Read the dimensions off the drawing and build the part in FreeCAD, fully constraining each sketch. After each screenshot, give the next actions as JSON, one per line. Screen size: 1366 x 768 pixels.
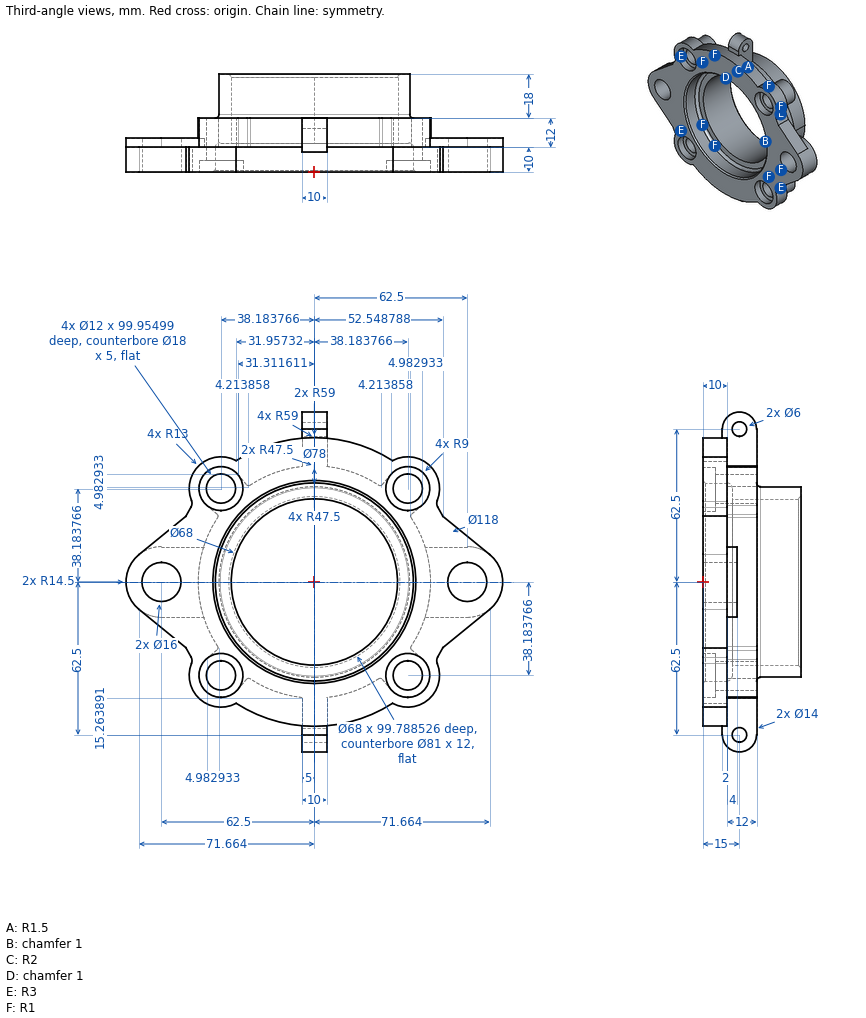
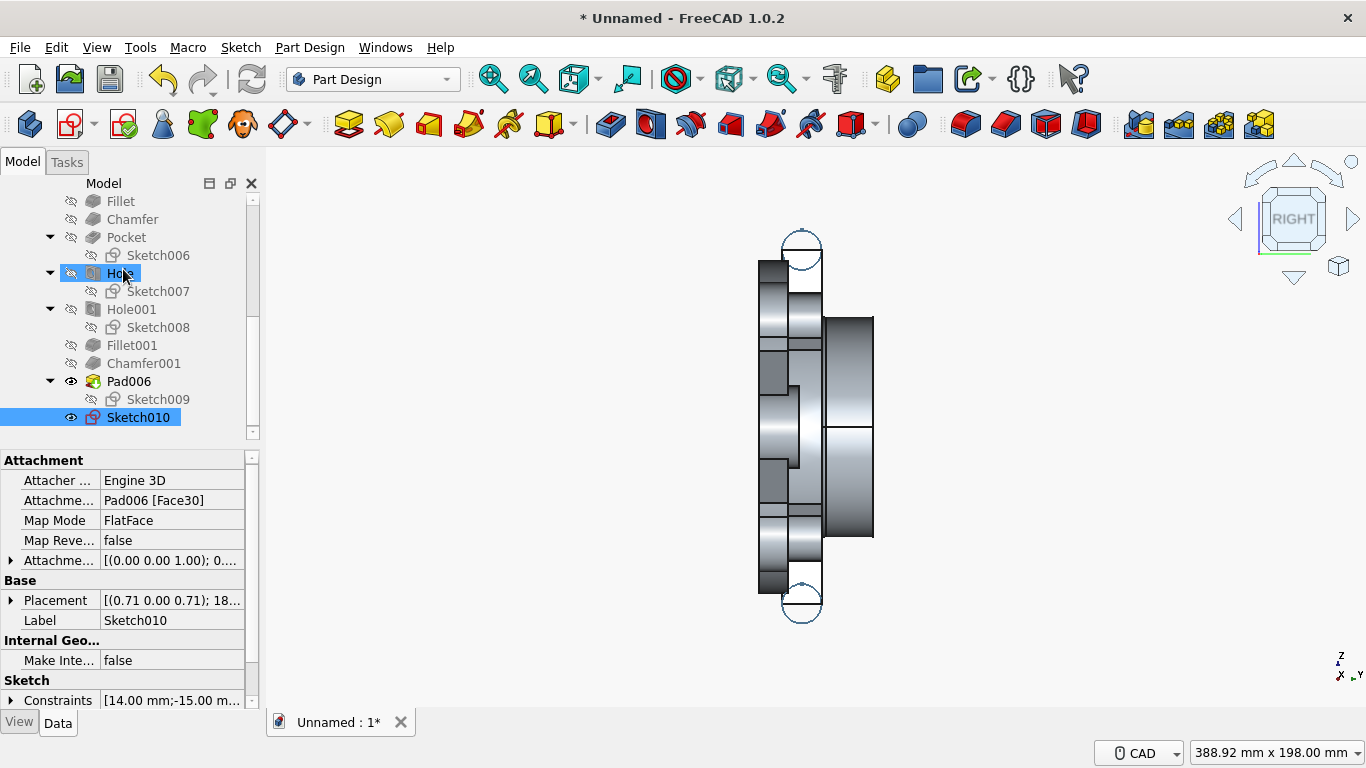
{"action": "left_click", "coordinate": [350, 124]}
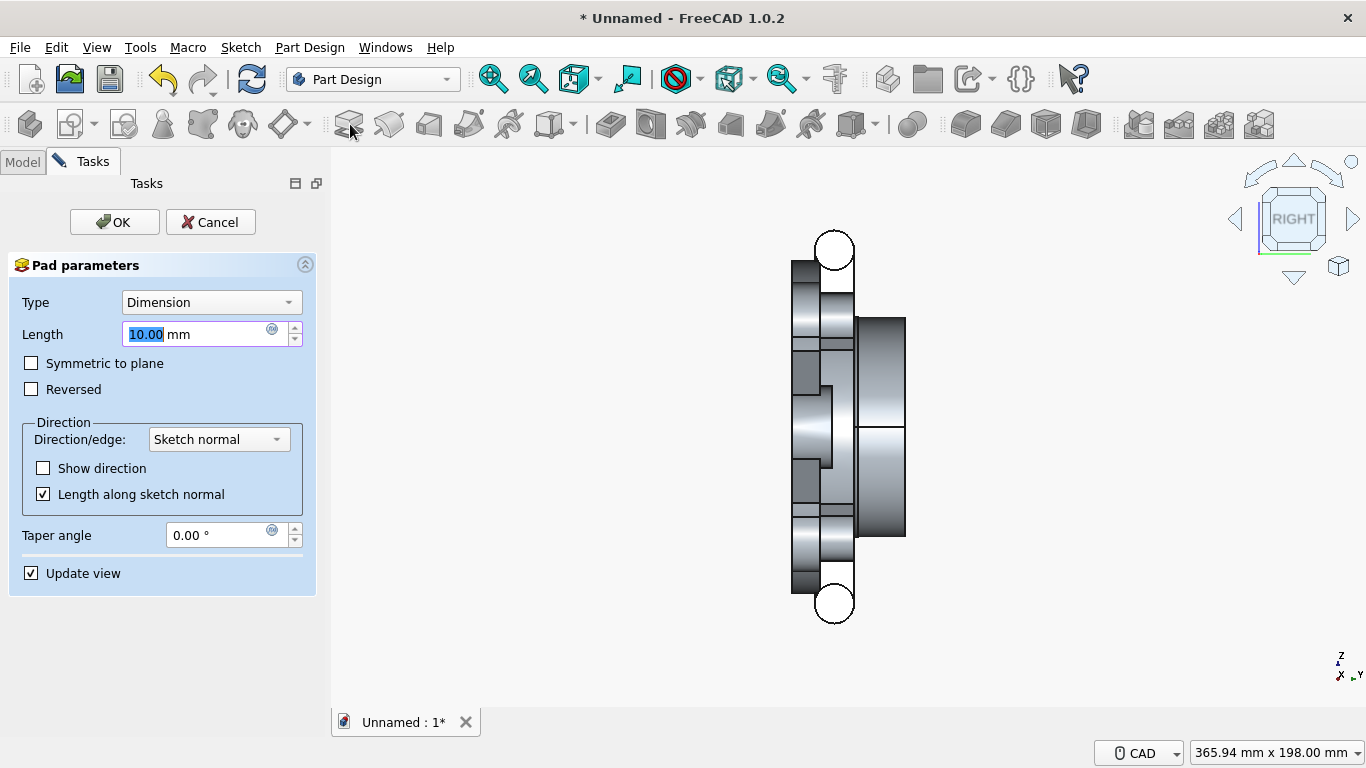
{"action": "type", "text": "10"}
{"action": "key", "text": "Tab"}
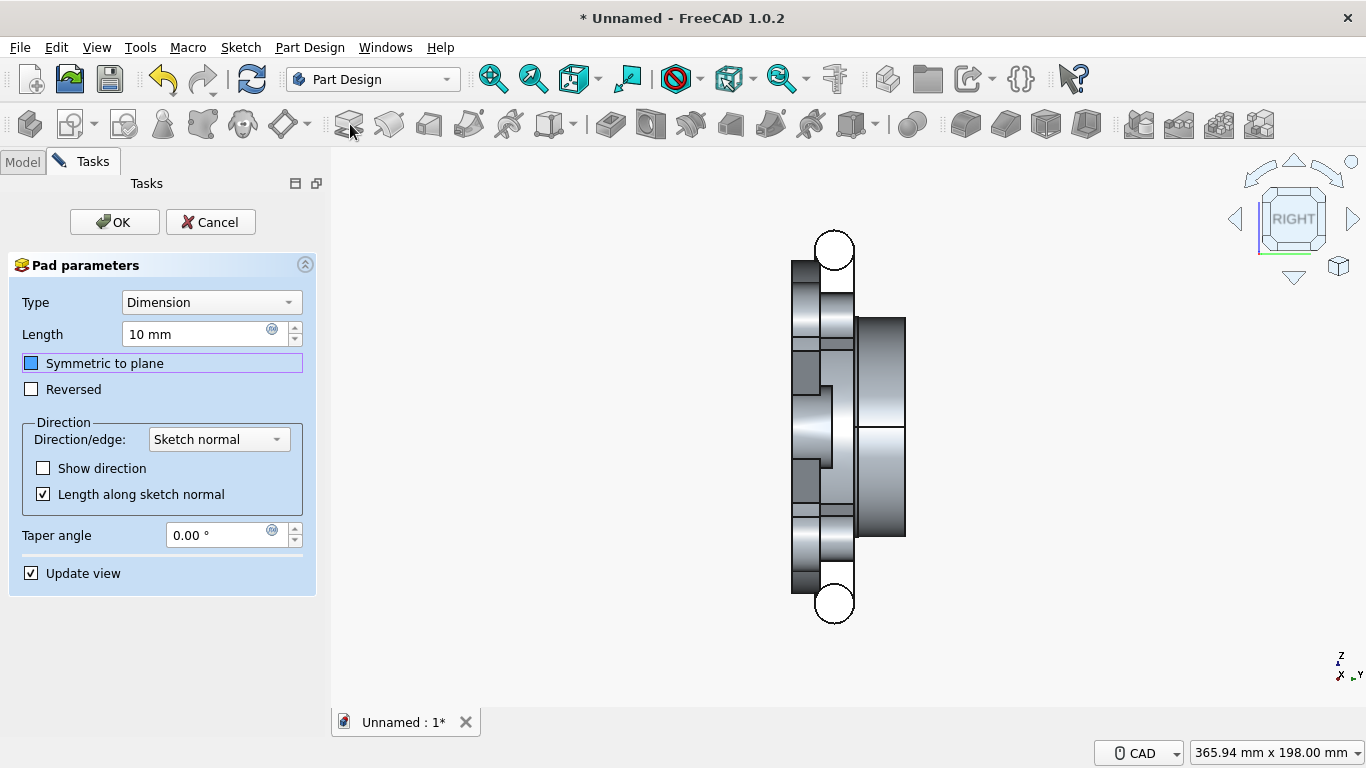
{"action": "left_click", "coordinate": [30, 389]}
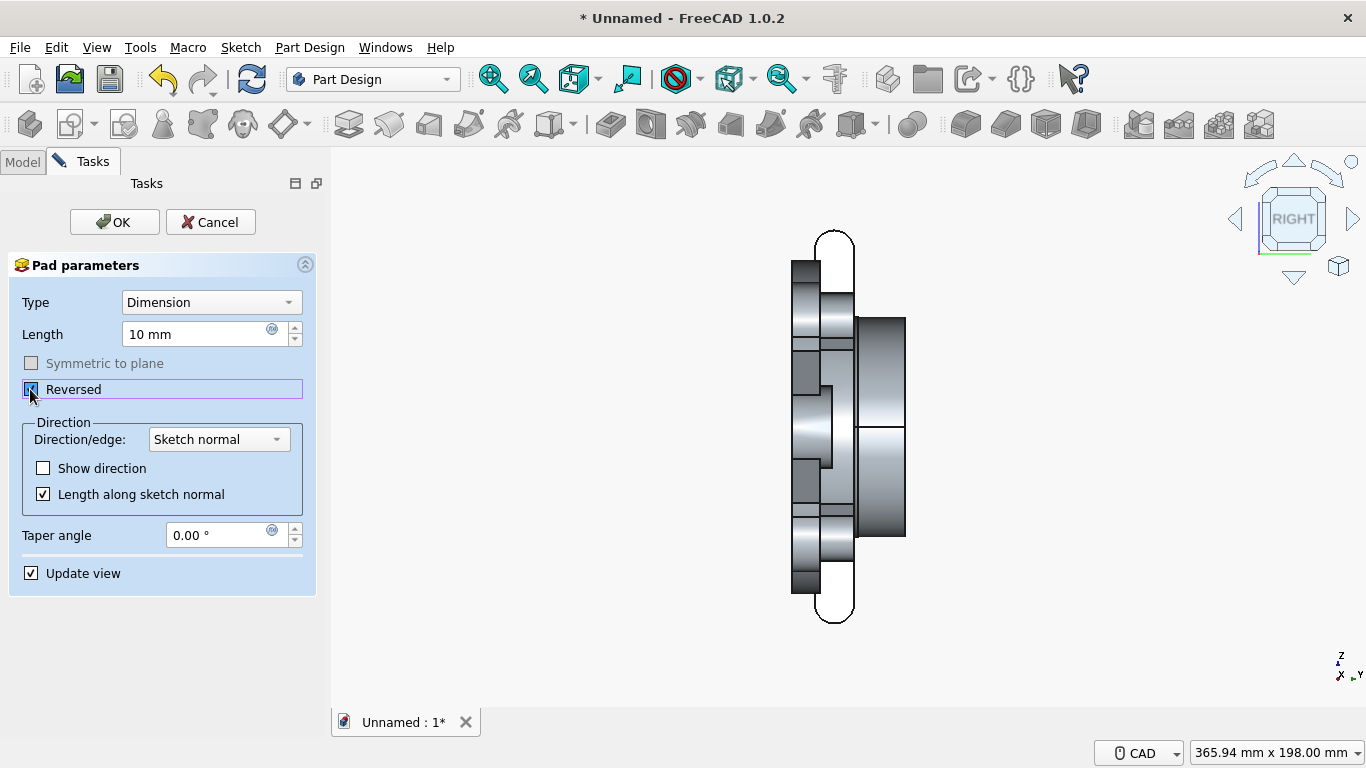
{"action": "left_click", "coordinate": [115, 222]}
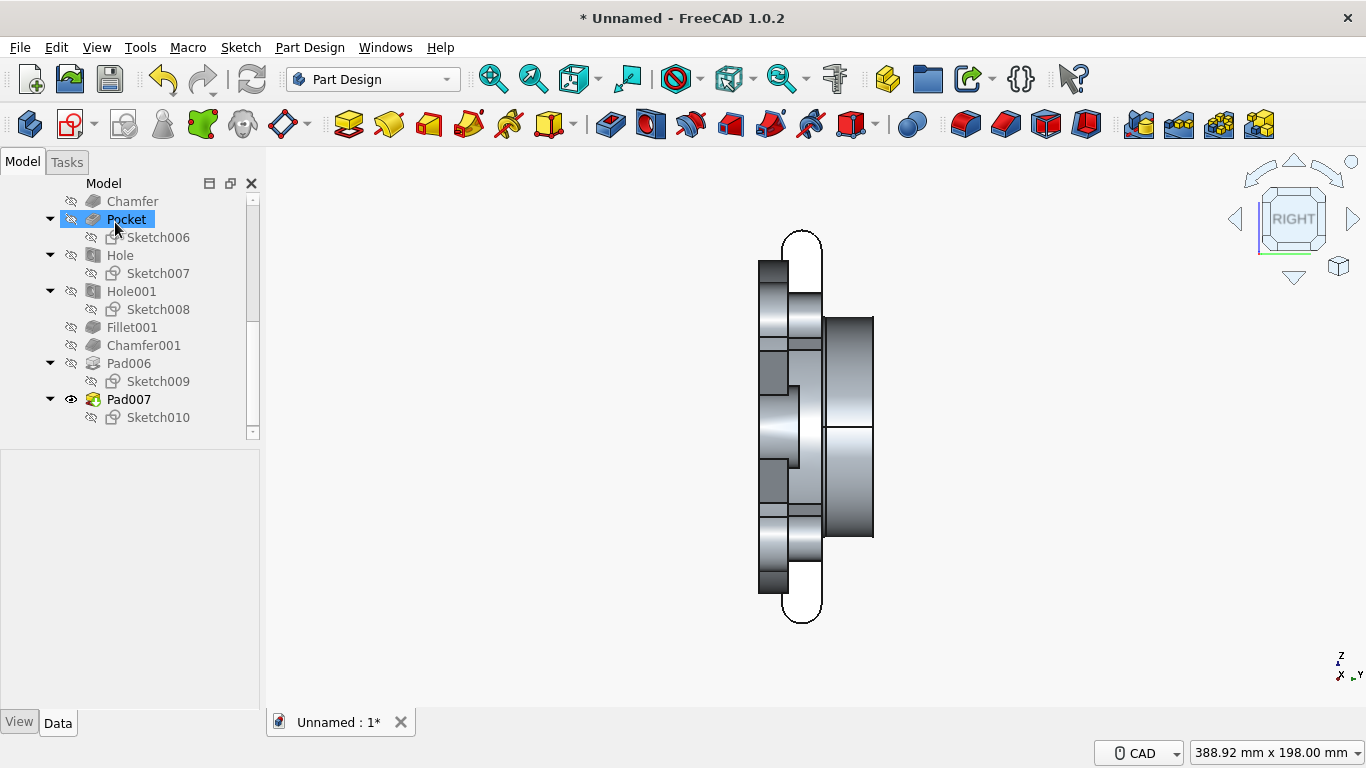
{"action": "left_click", "coordinate": [802, 252]}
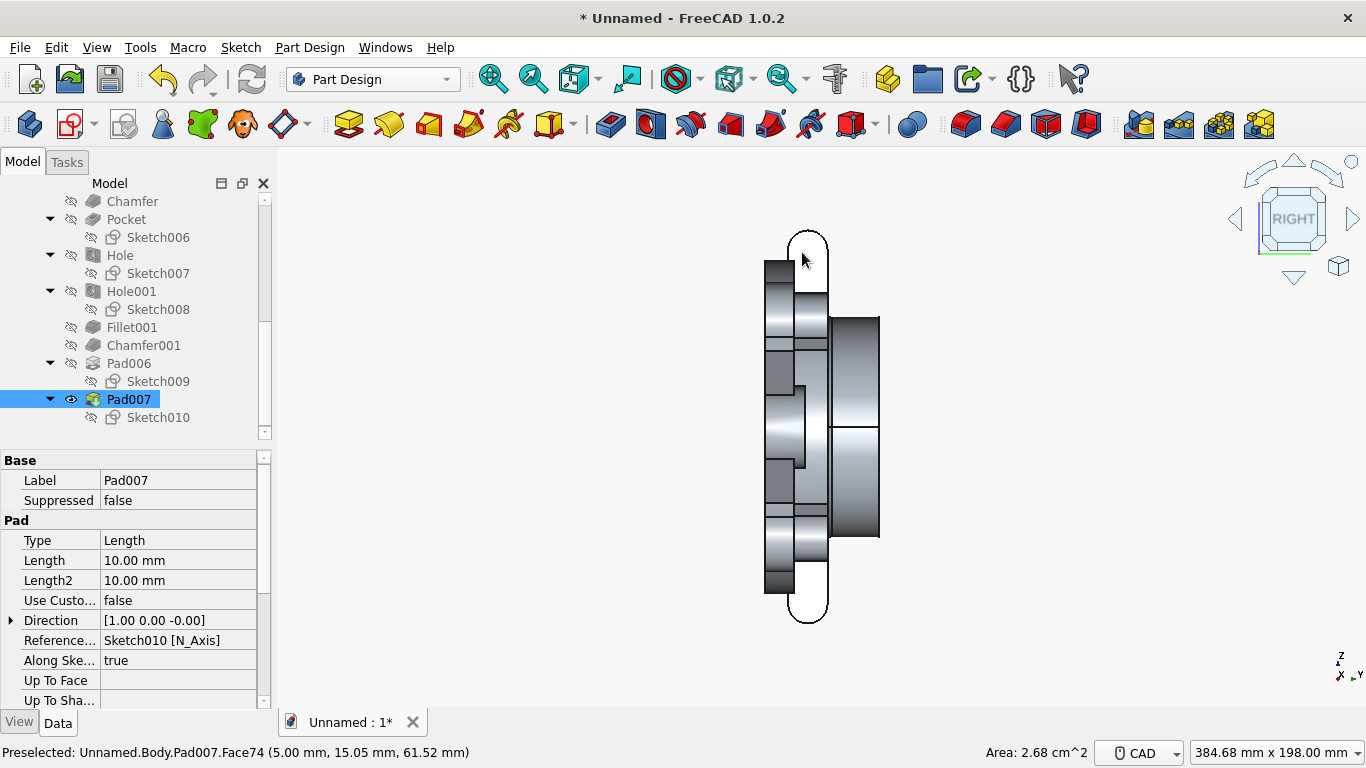
{"action": "left_click", "coordinate": [70, 124]}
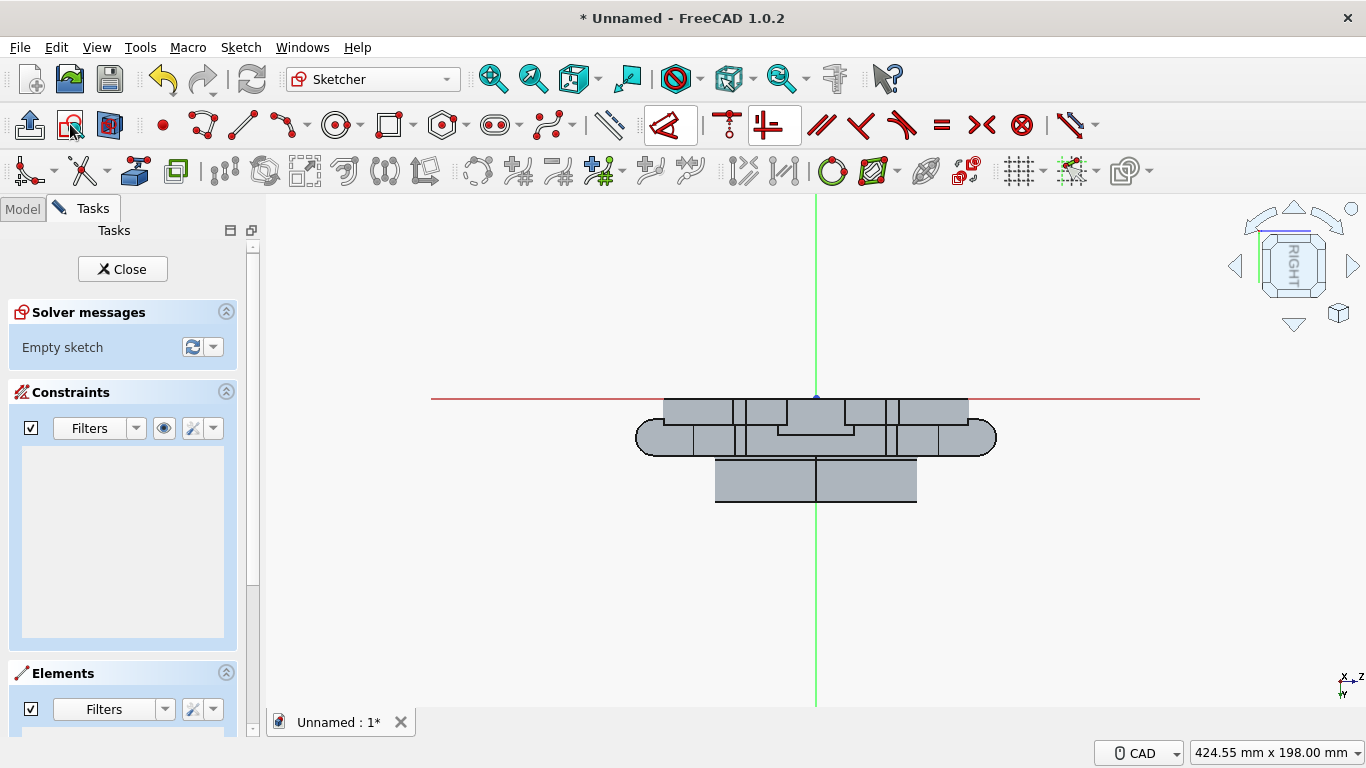
{"action": "left_click", "coordinate": [110, 126]}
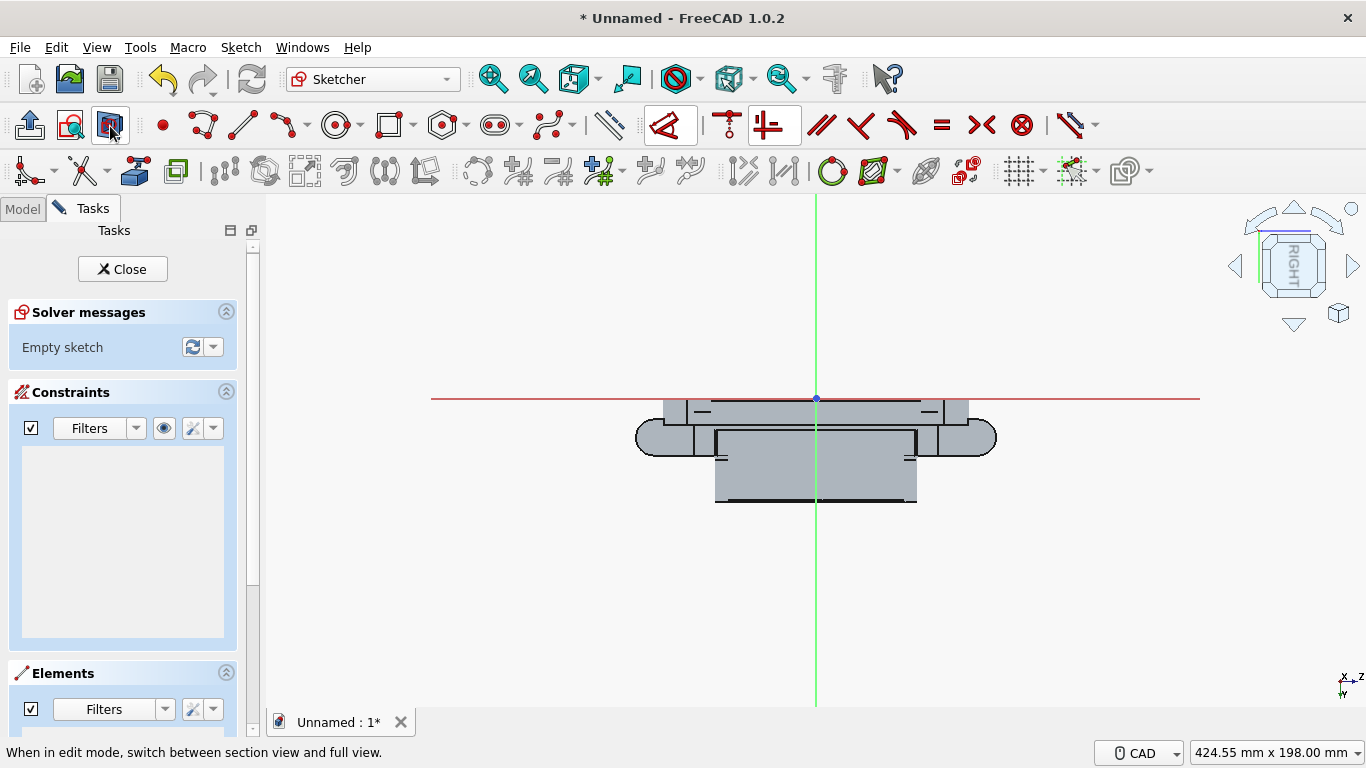
{"action": "scroll", "coordinate": [899, 387], "scroll_direction": "up", "scroll_amount": 3}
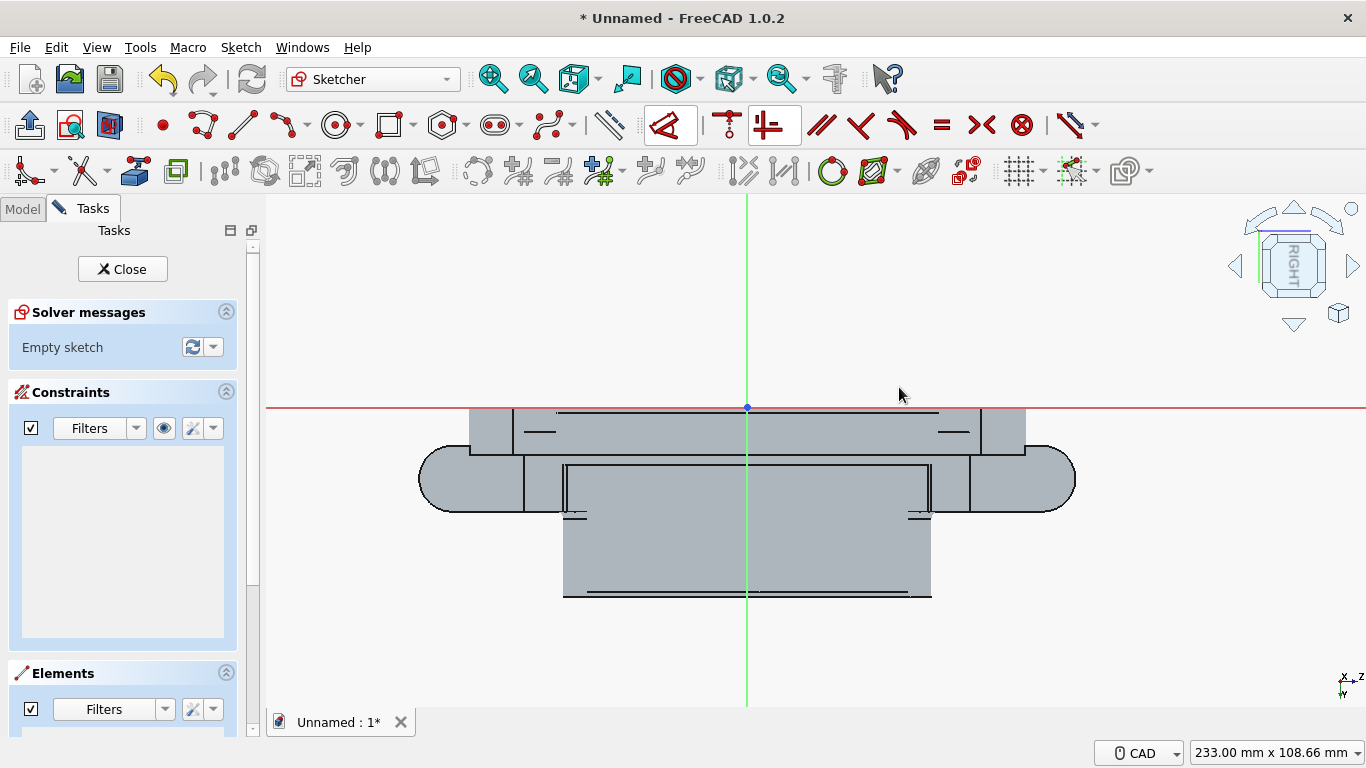
{"action": "left_click", "coordinate": [336, 126]}